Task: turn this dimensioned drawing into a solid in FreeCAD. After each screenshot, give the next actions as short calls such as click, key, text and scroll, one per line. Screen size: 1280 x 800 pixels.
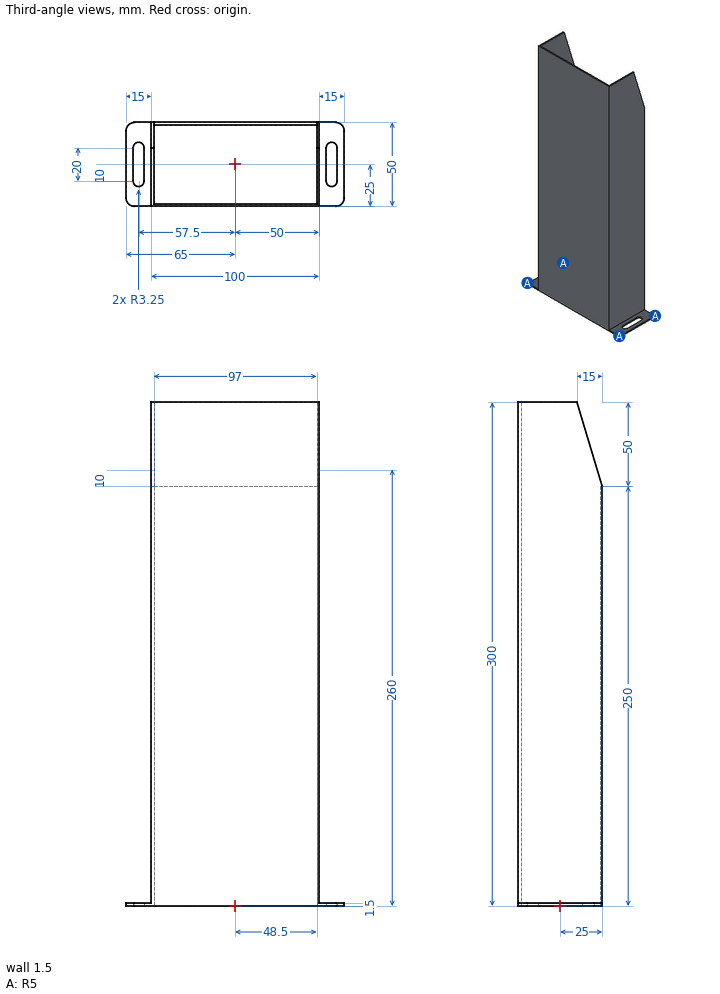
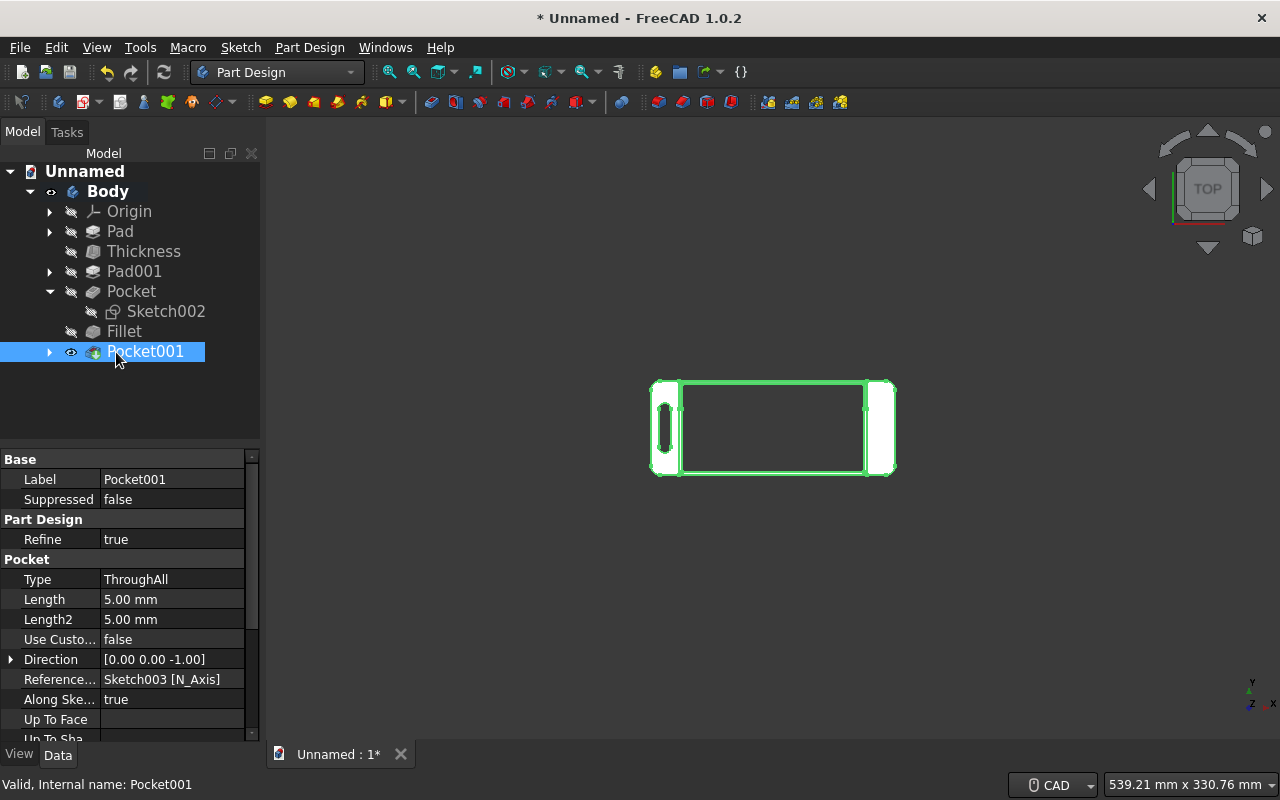
click(768, 102)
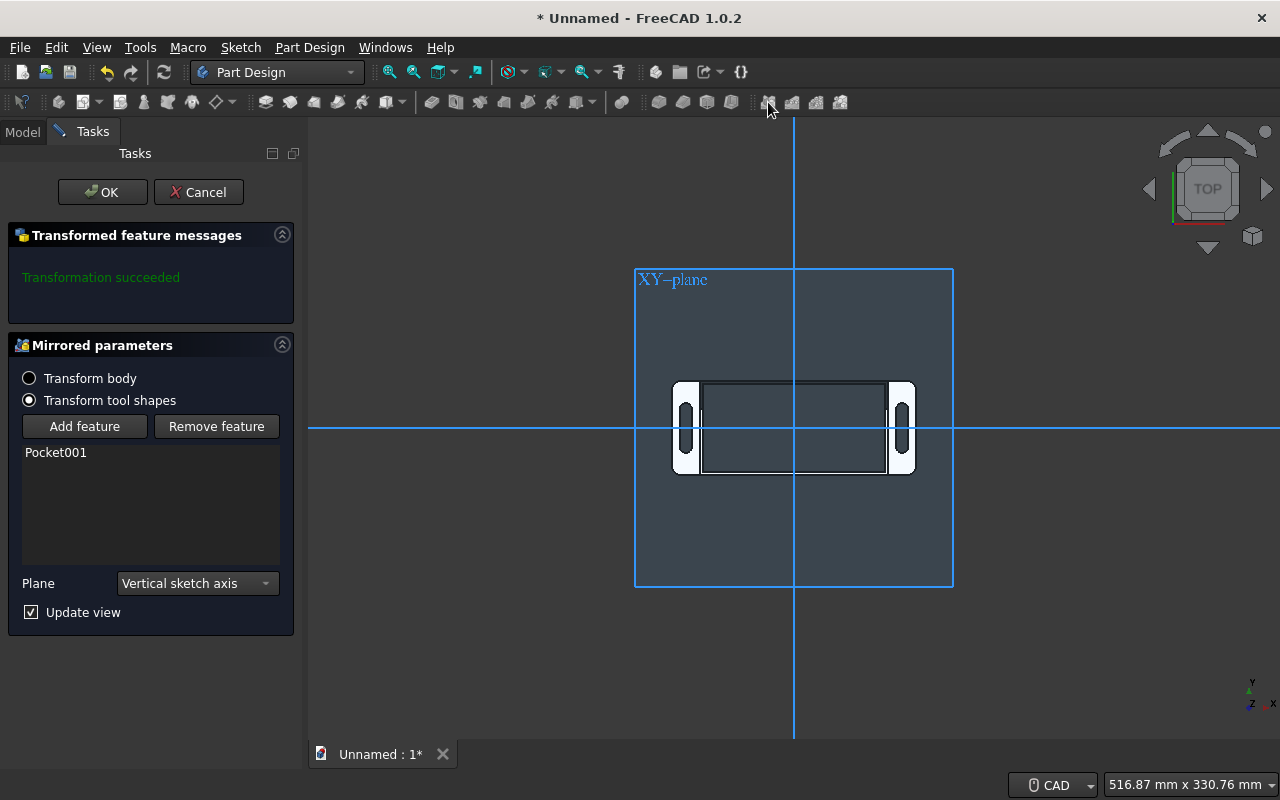
click(198, 584)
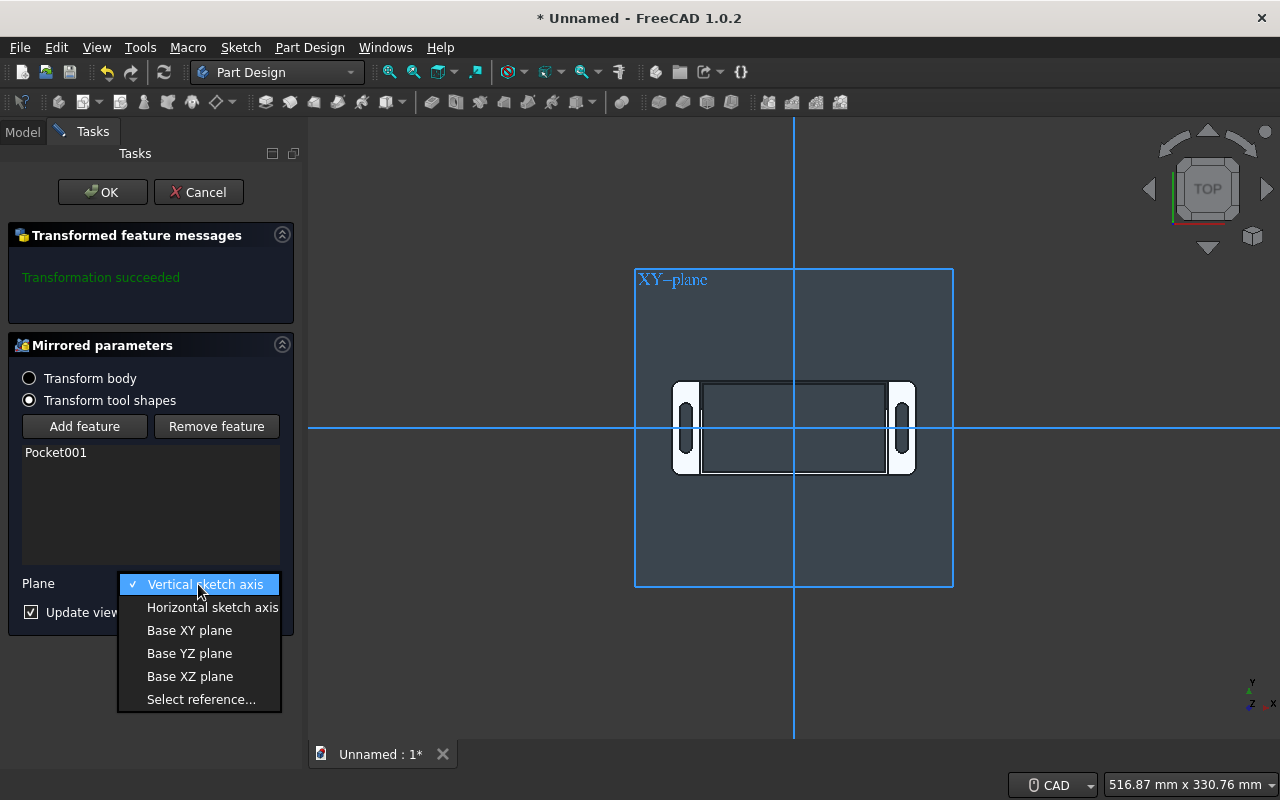
click(198, 654)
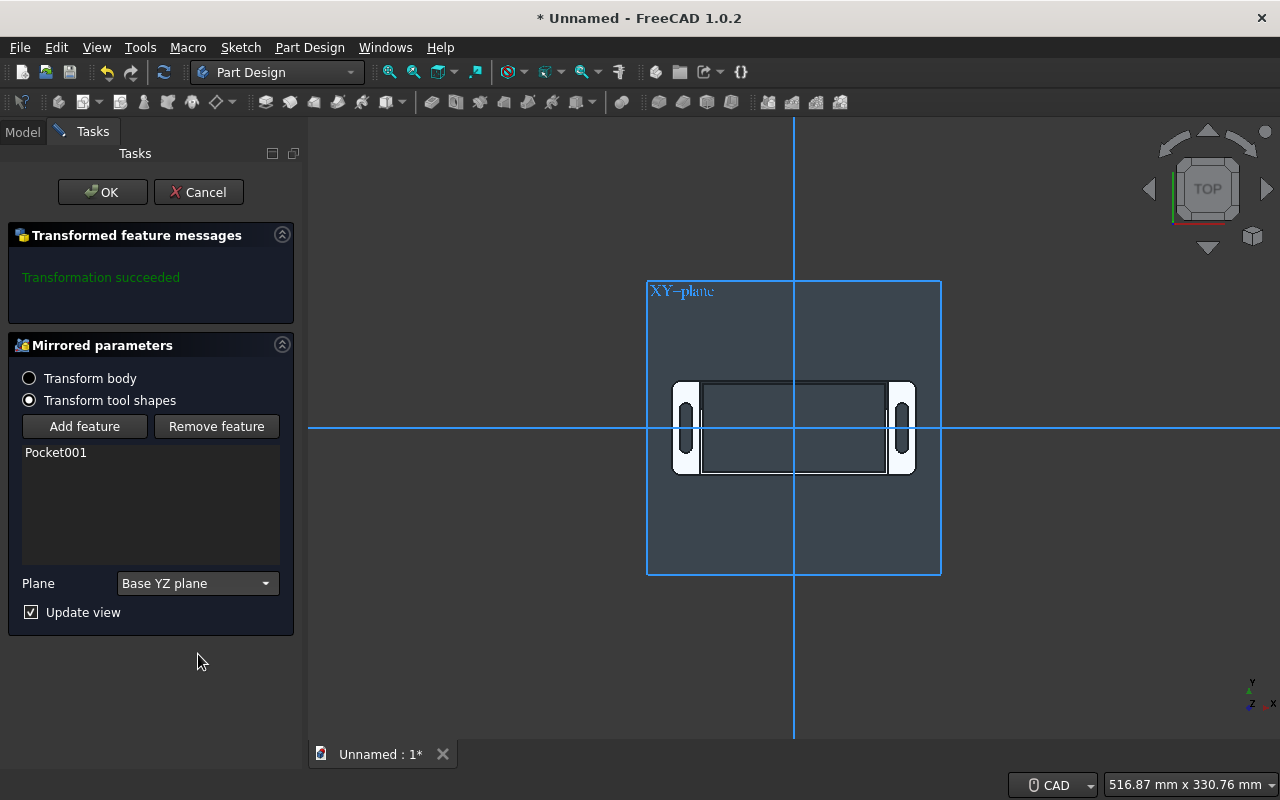
click(103, 192)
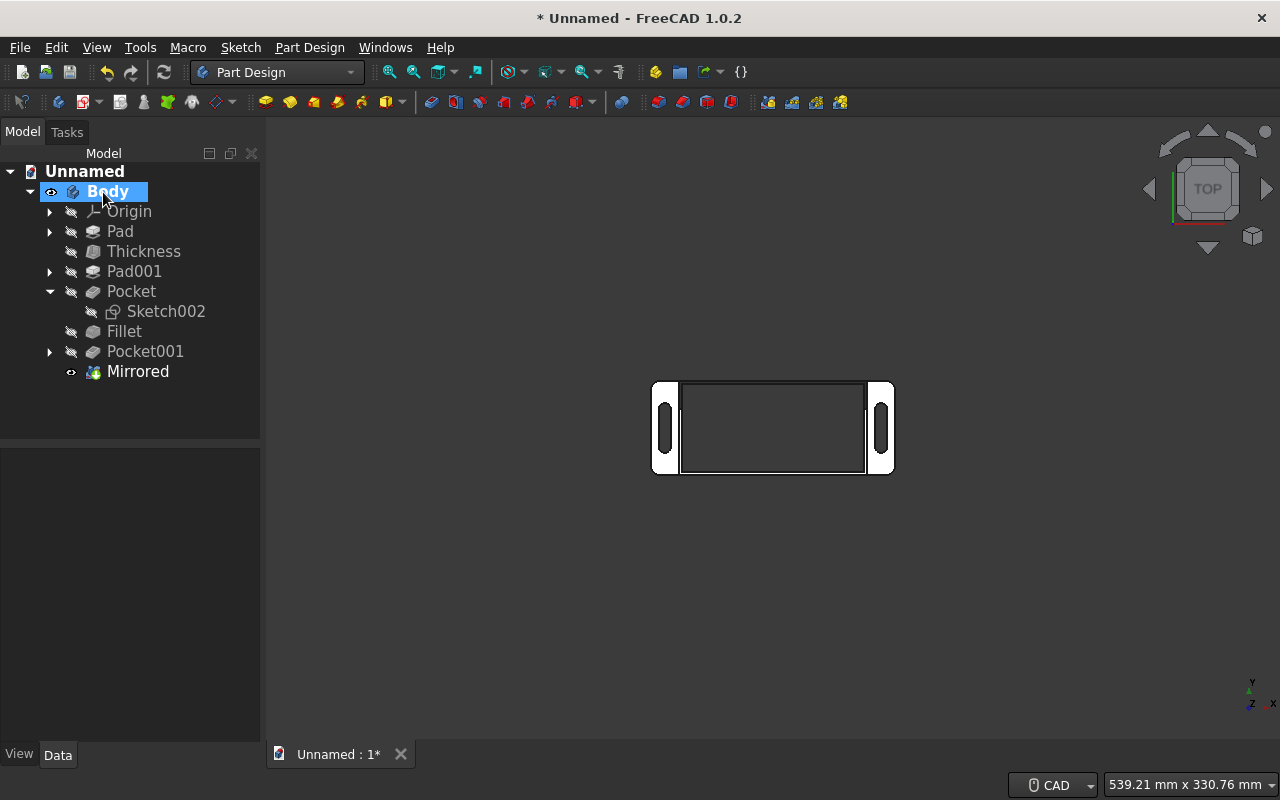
click(390, 72)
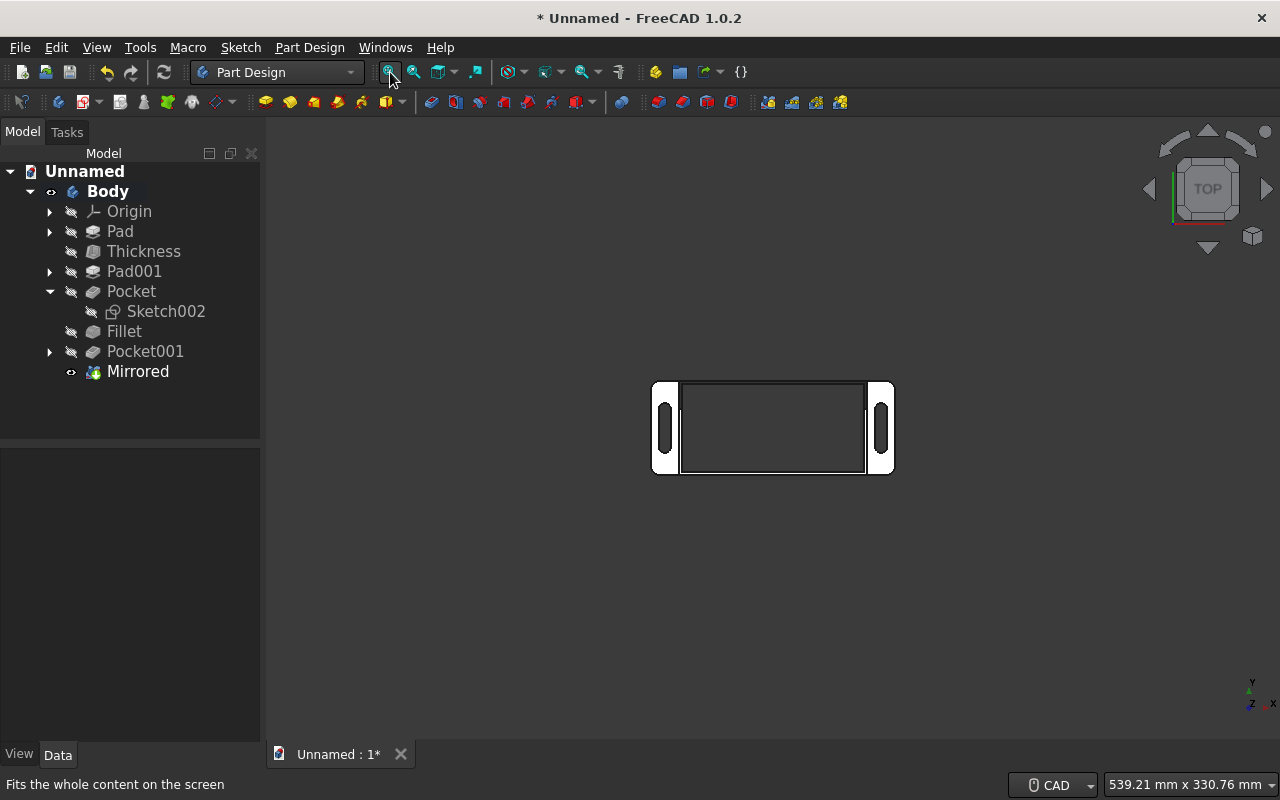
key(4)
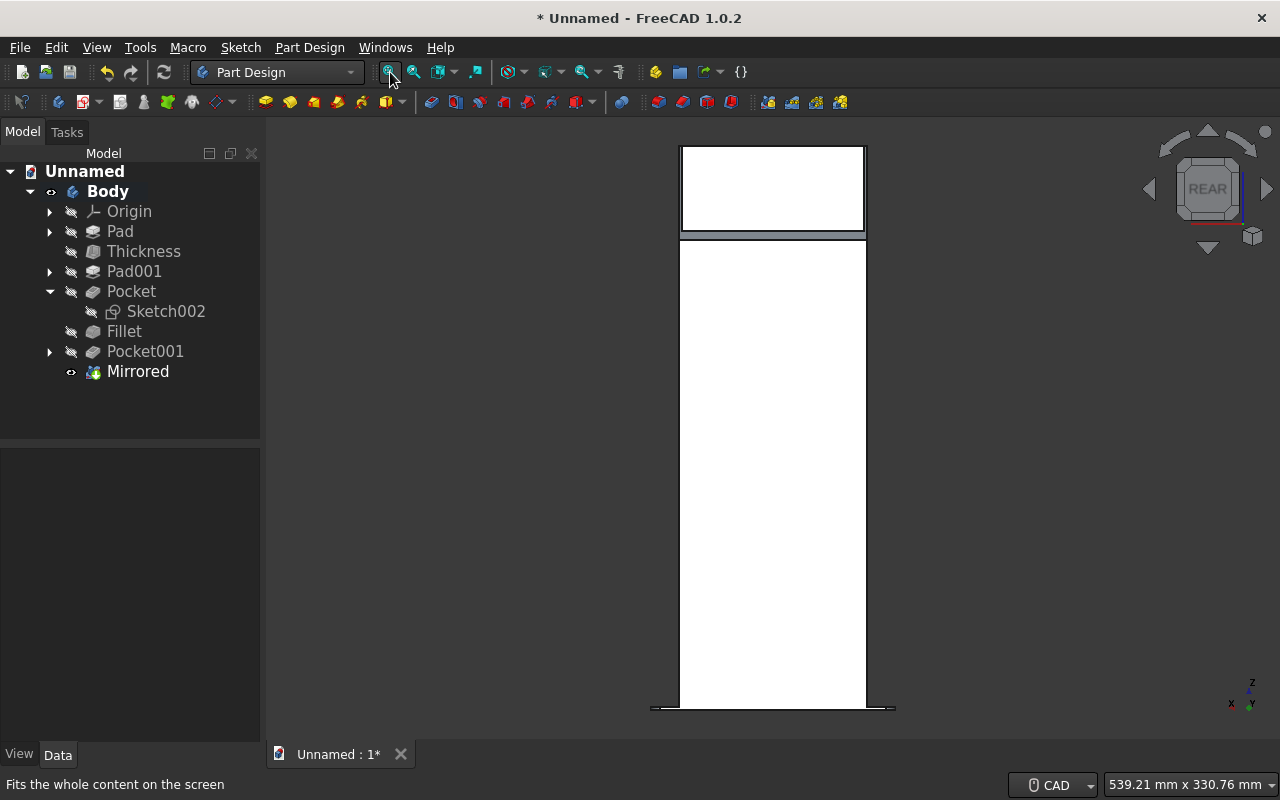
click(773, 340)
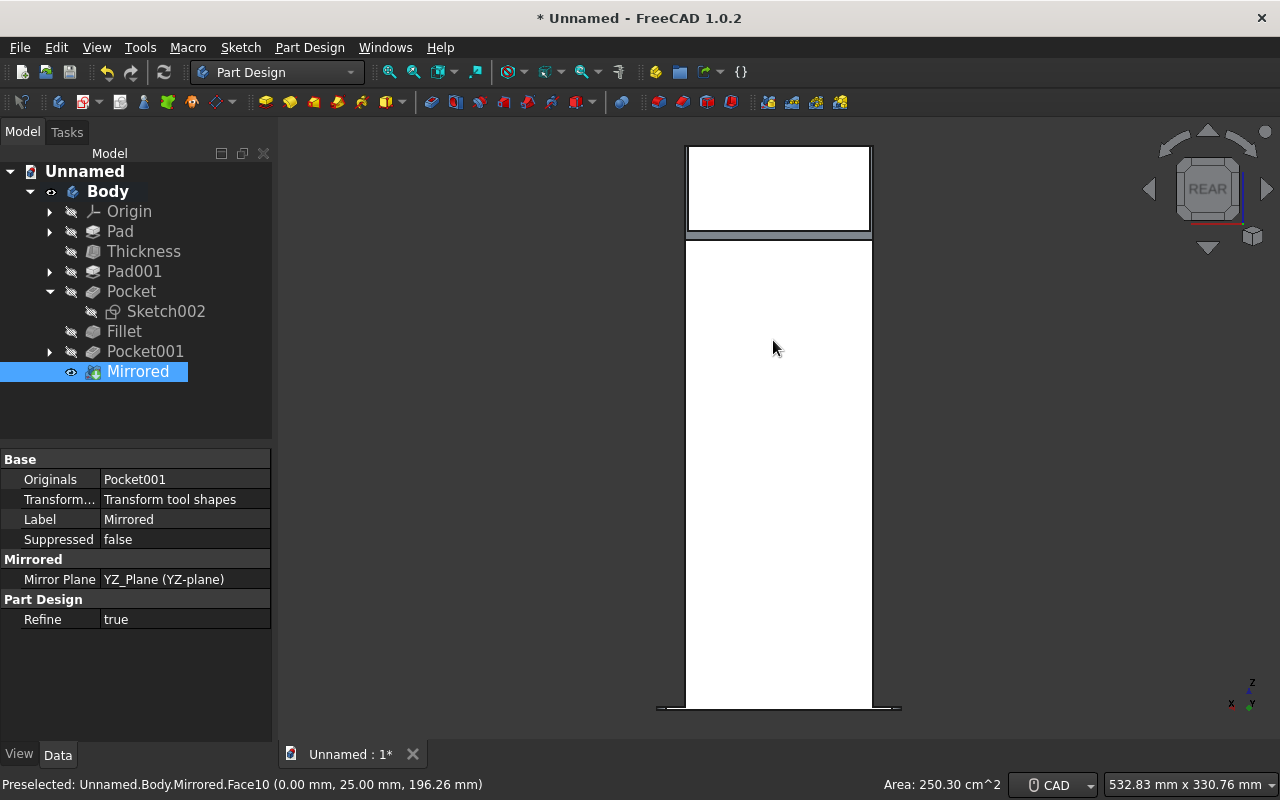
click(84, 102)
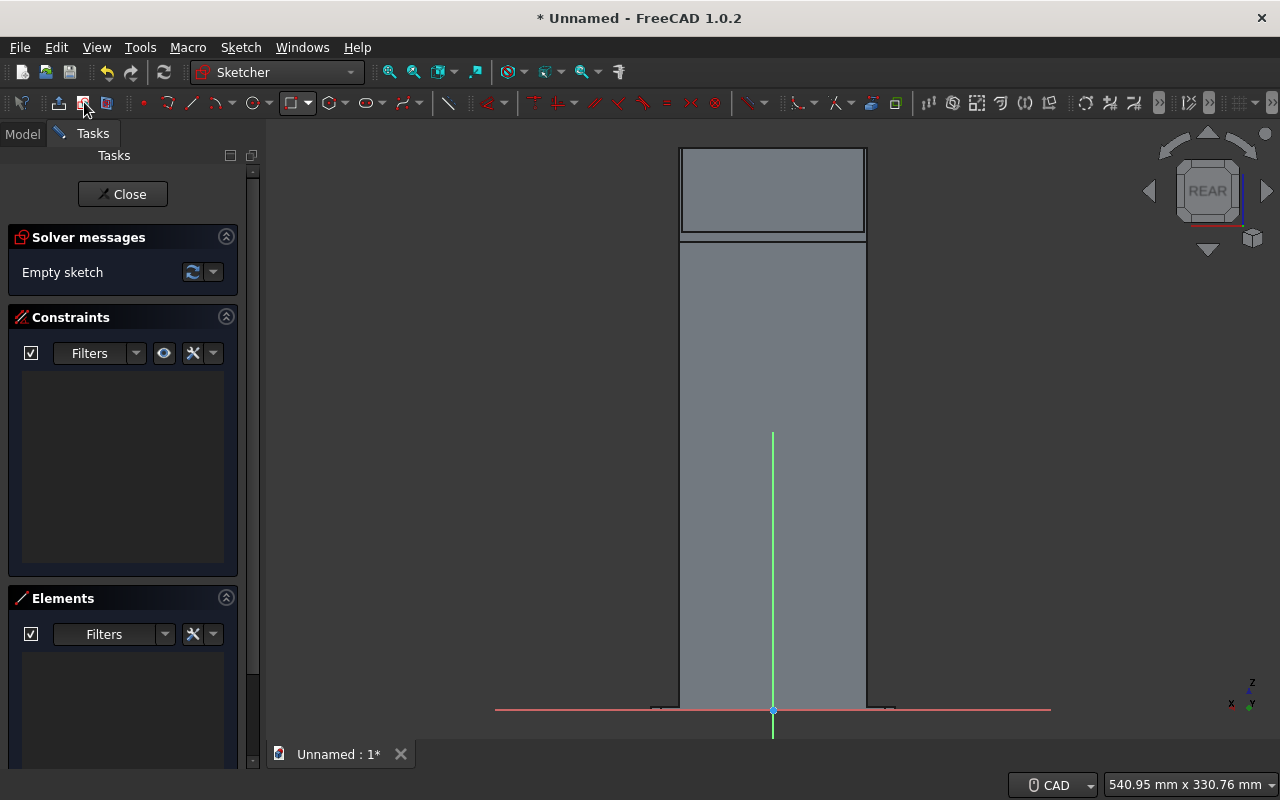
scroll(803, 147, up, 6)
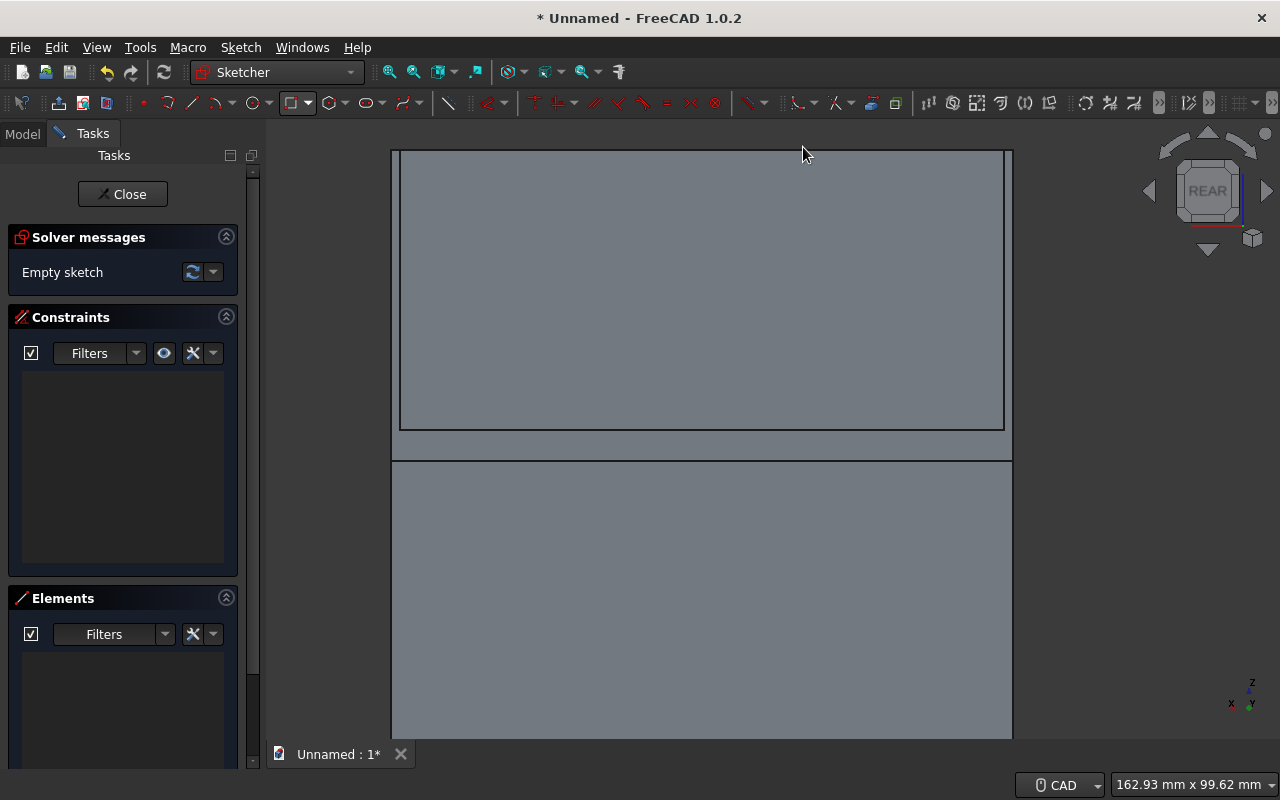
click(292, 104)